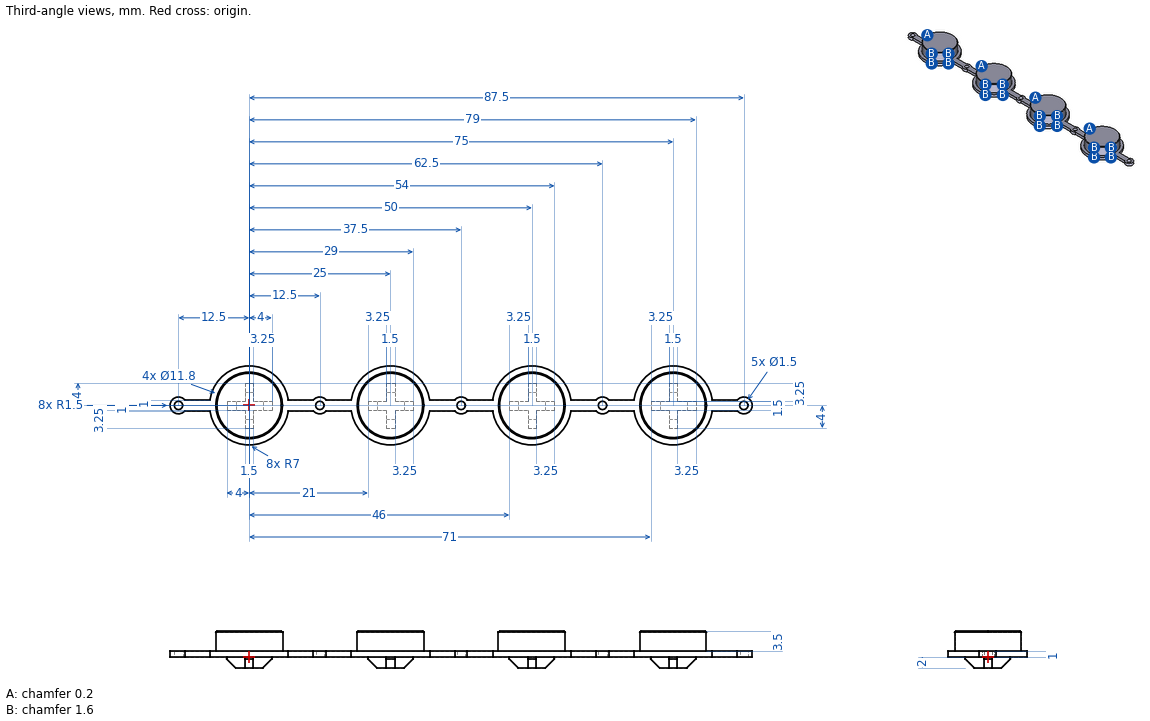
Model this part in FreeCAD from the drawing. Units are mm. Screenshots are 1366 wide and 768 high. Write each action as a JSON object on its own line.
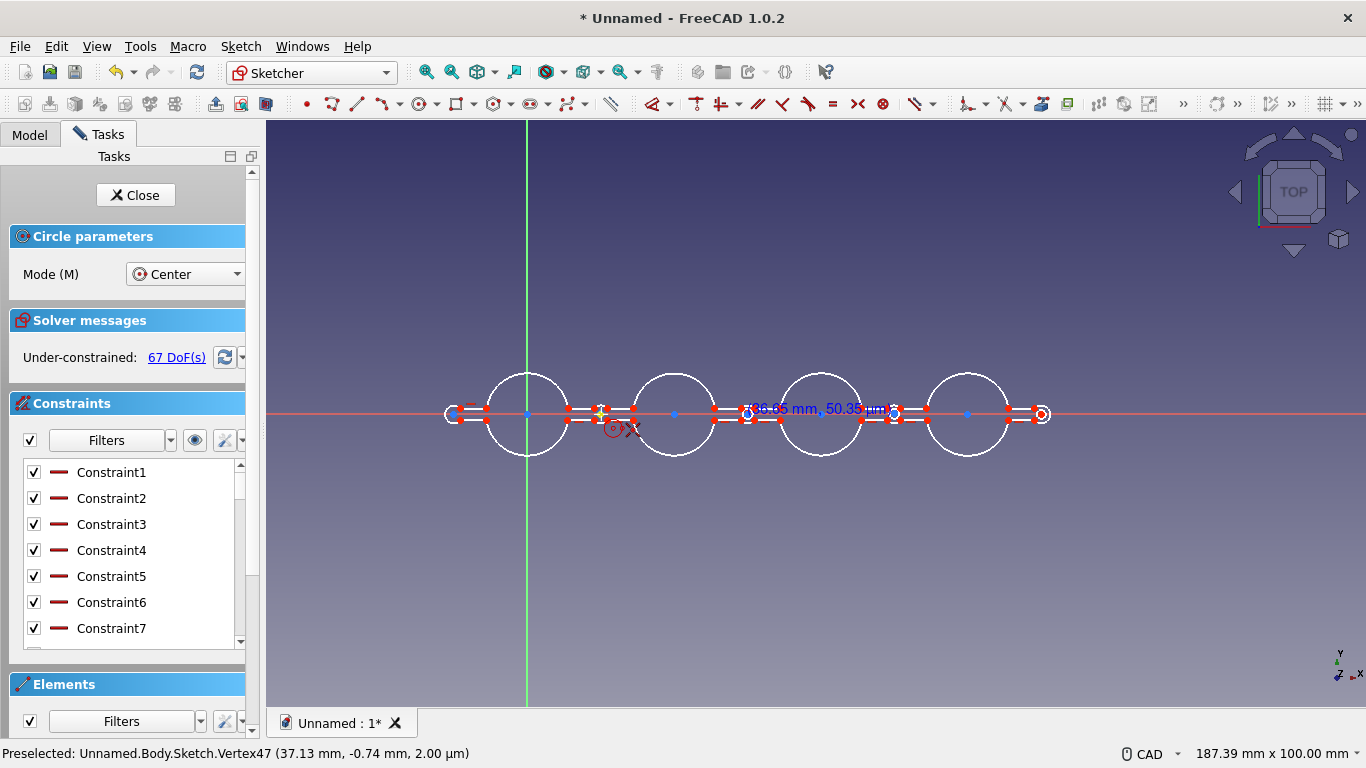
{"action": "scroll", "coordinate": [601, 414], "scroll_direction": "up", "scroll_amount": 3}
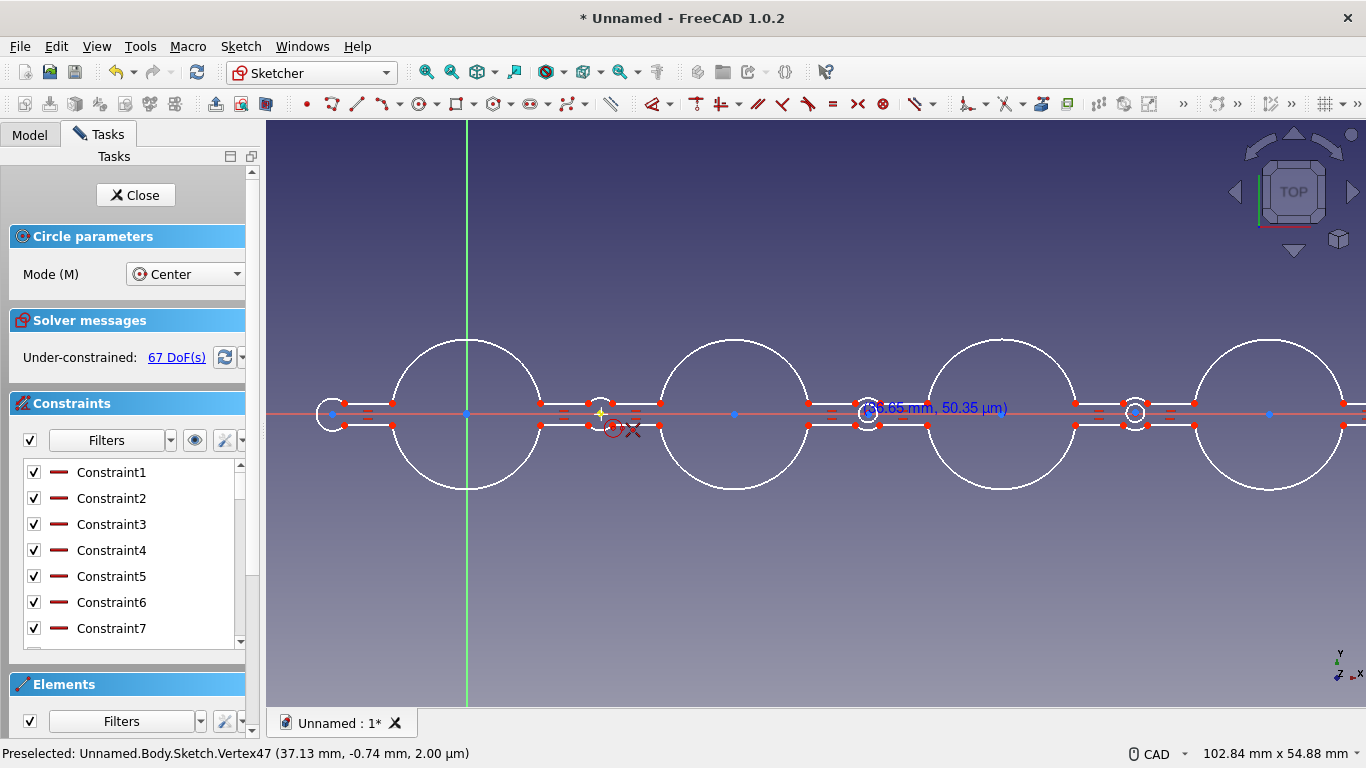
{"action": "left_click", "coordinate": [601, 414]}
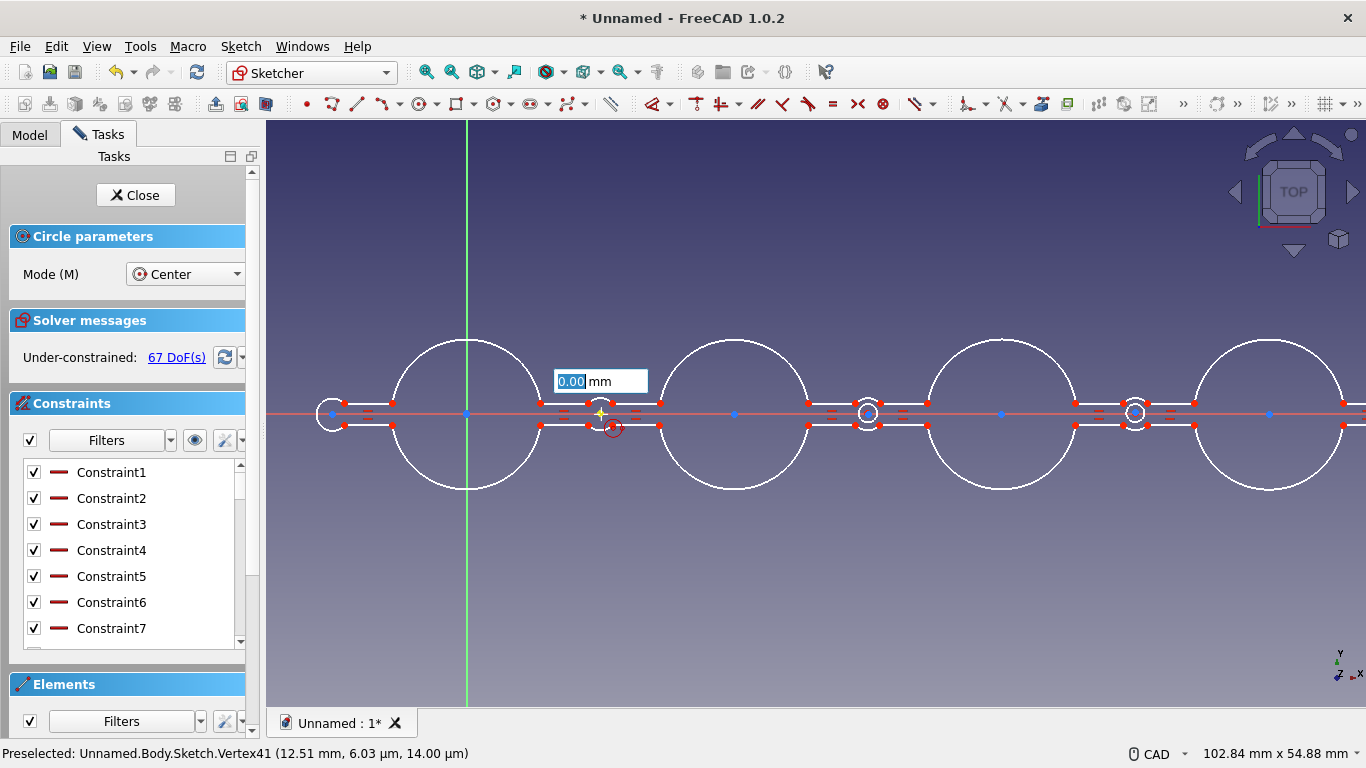
{"action": "scroll", "coordinate": [598, 421], "scroll_direction": "up", "scroll_amount": 4}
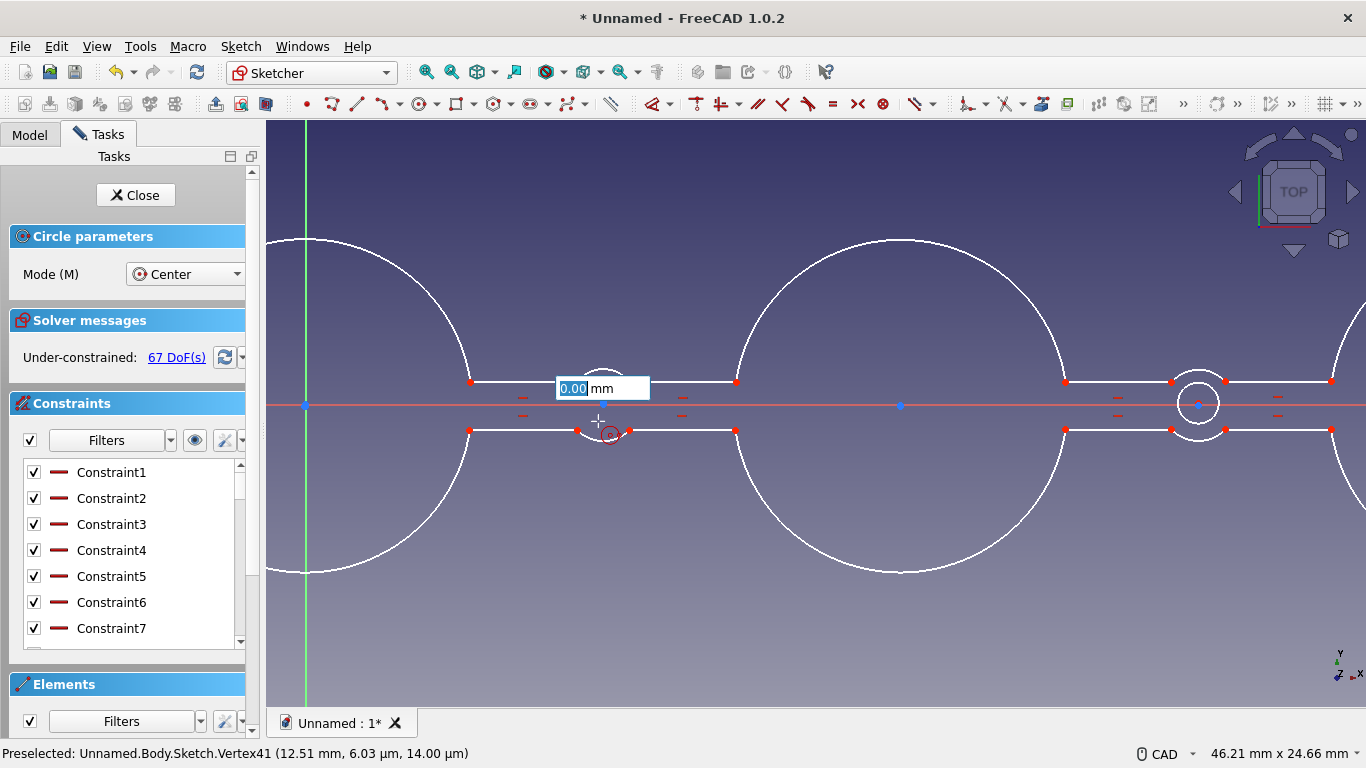
{"action": "left_click", "coordinate": [597, 421]}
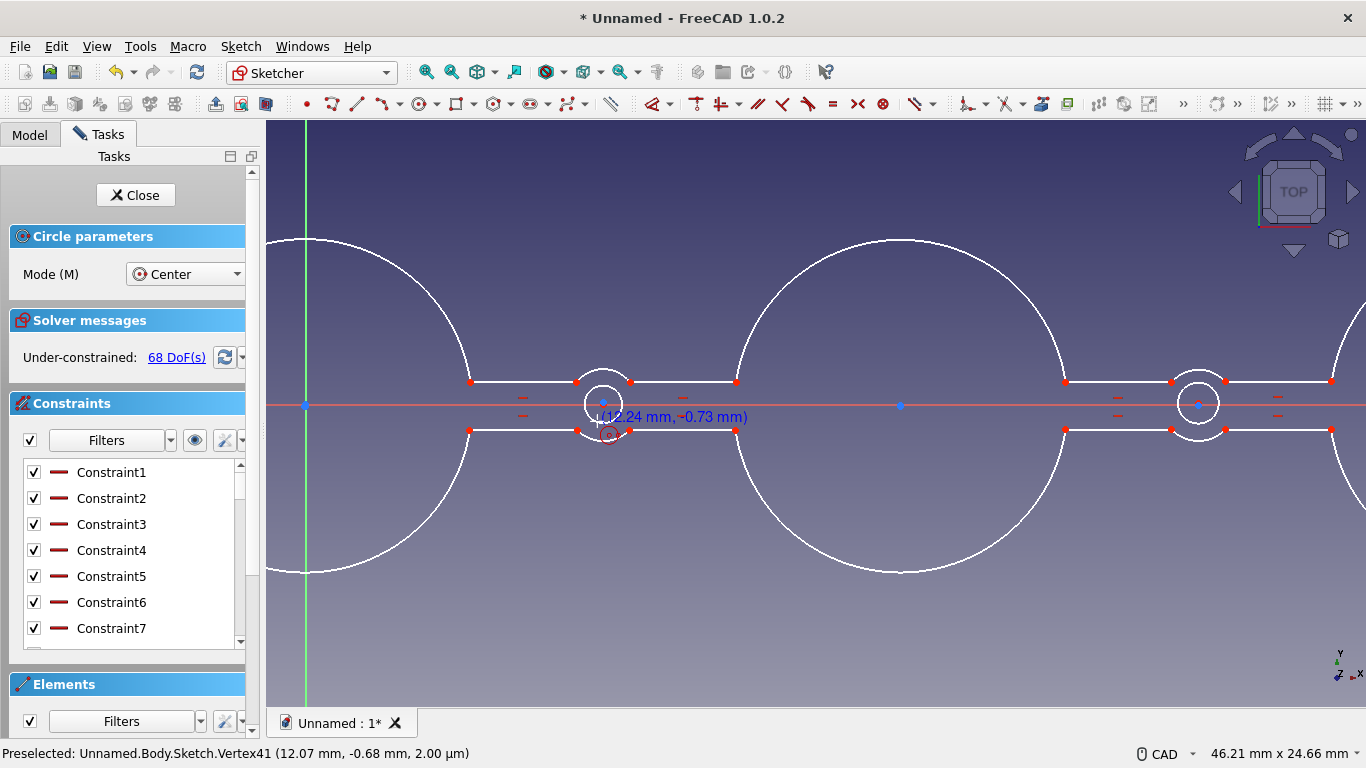
{"action": "scroll", "coordinate": [600, 416], "scroll_direction": "down", "scroll_amount": 7}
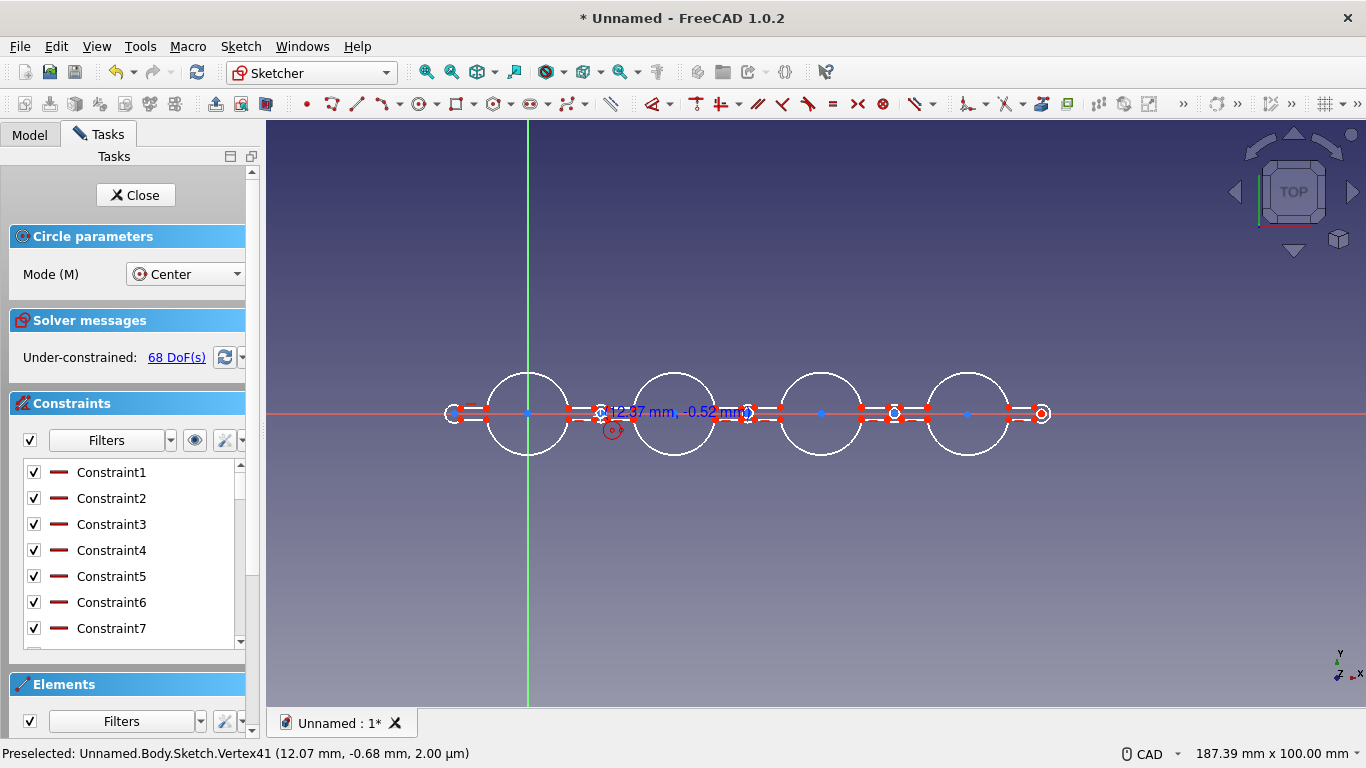
{"action": "scroll", "coordinate": [454, 414], "scroll_direction": "up", "scroll_amount": 9}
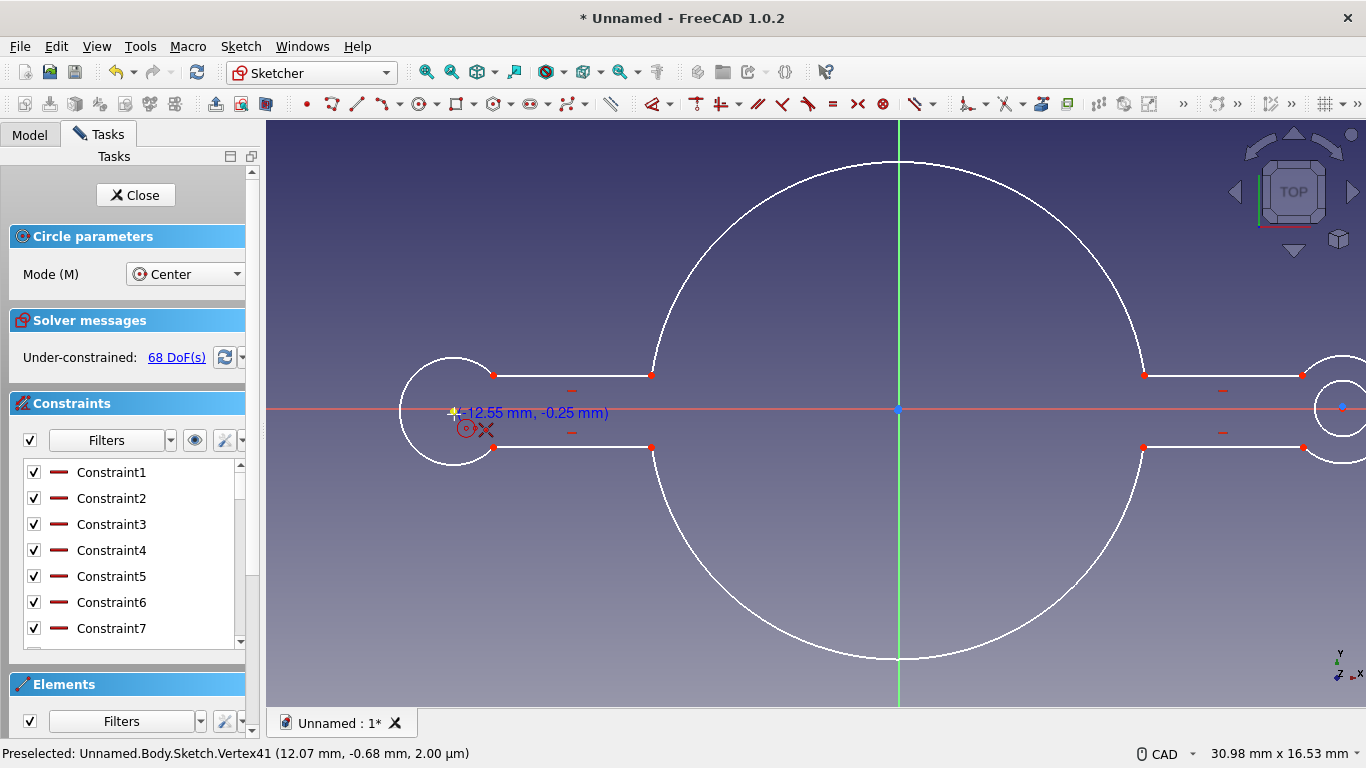
{"action": "scroll", "coordinate": [454, 414], "scroll_direction": "down", "scroll_amount": 9}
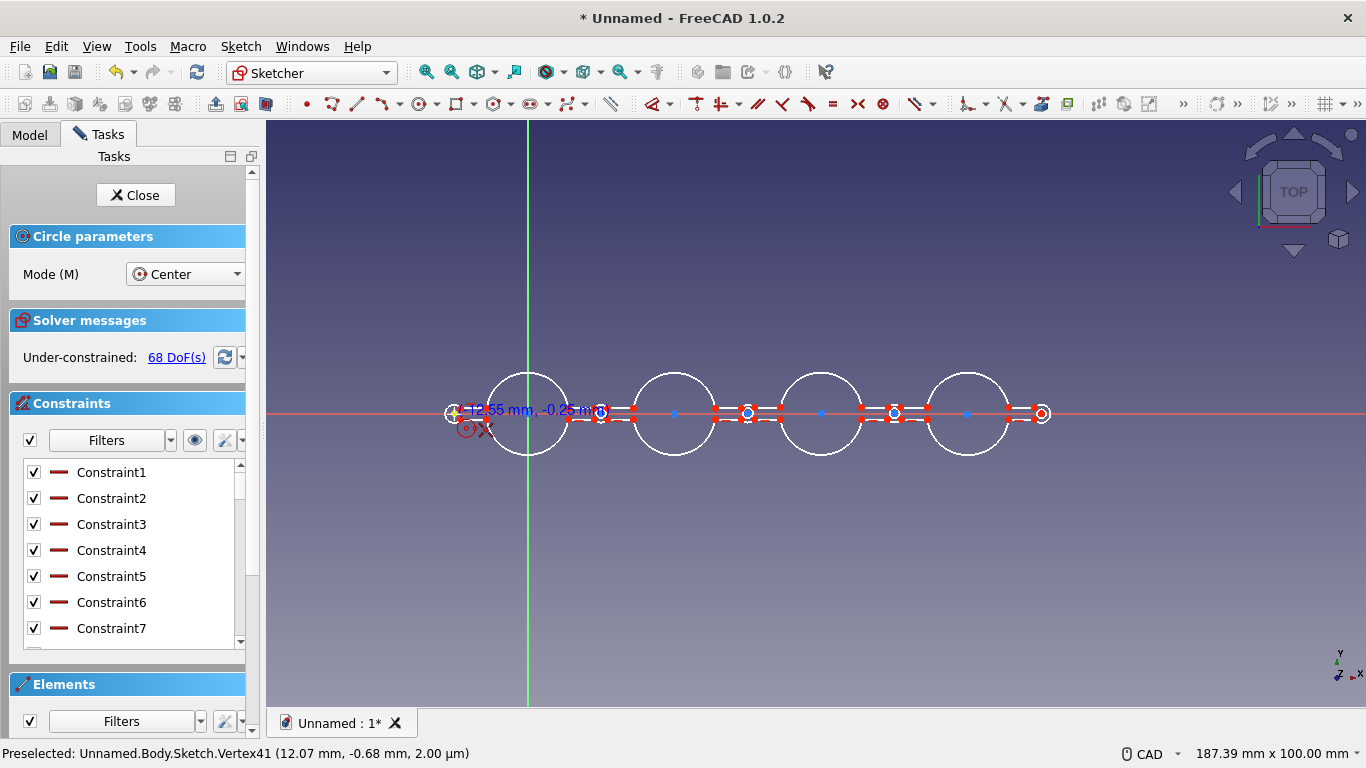
{"action": "scroll", "coordinate": [454, 414], "scroll_direction": "up", "scroll_amount": 3}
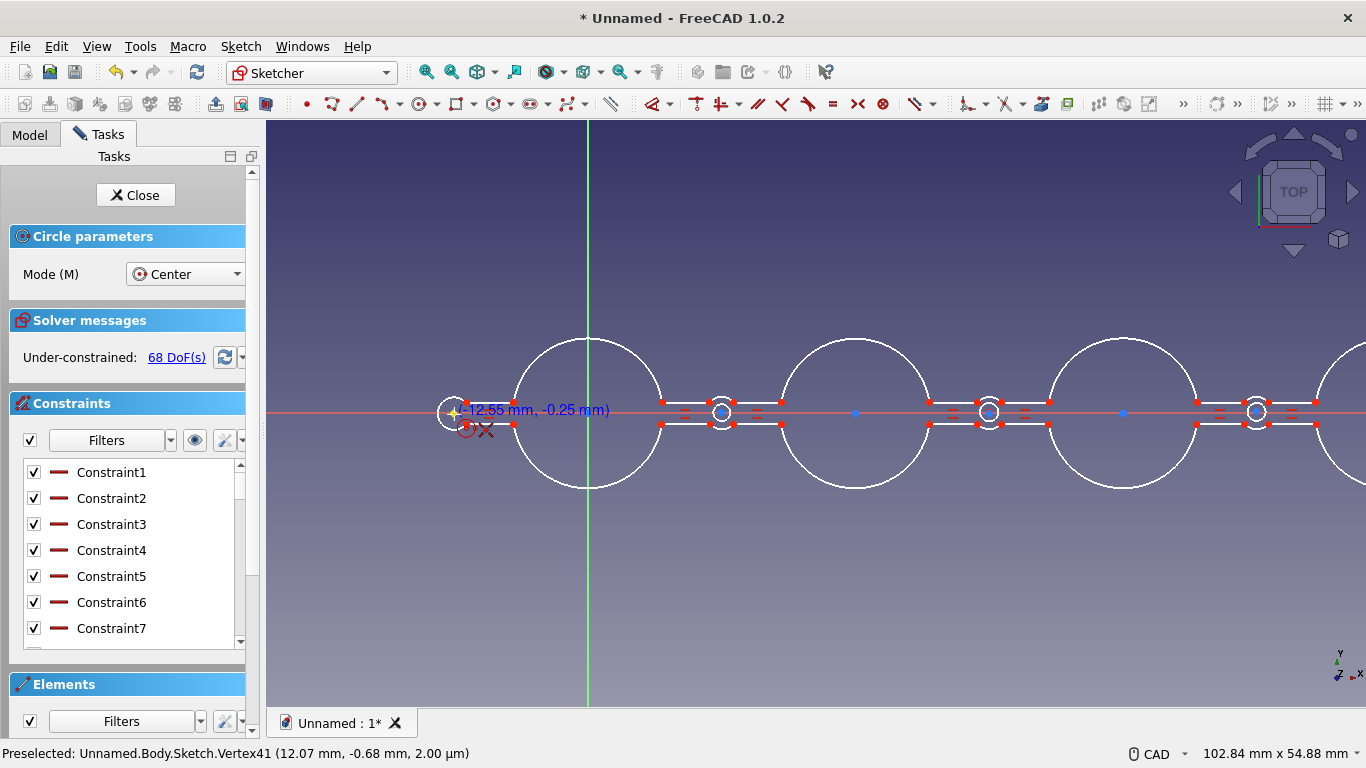
{"action": "left_click", "coordinate": [454, 413]}